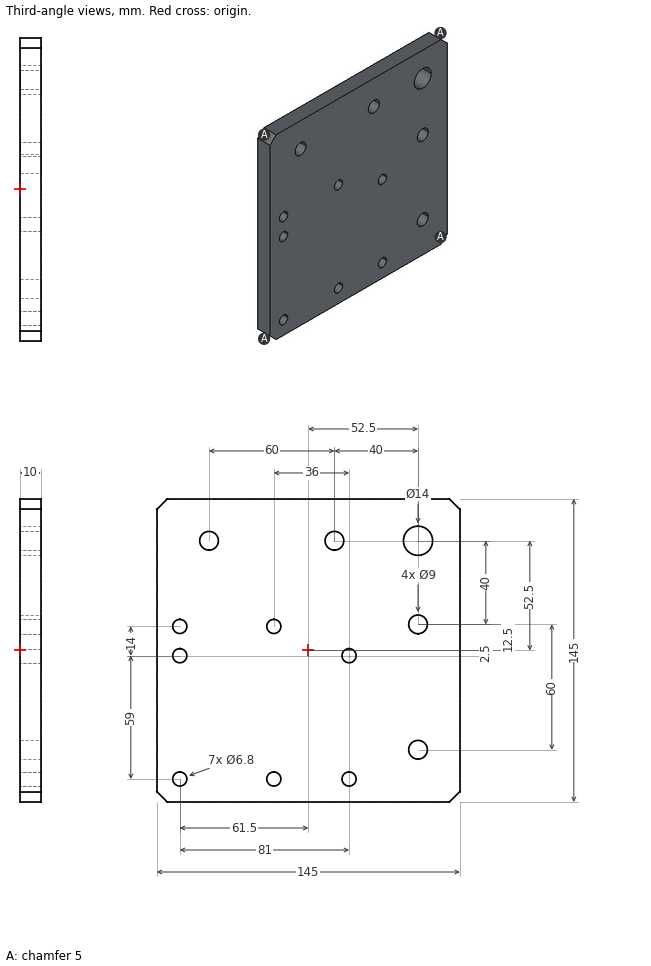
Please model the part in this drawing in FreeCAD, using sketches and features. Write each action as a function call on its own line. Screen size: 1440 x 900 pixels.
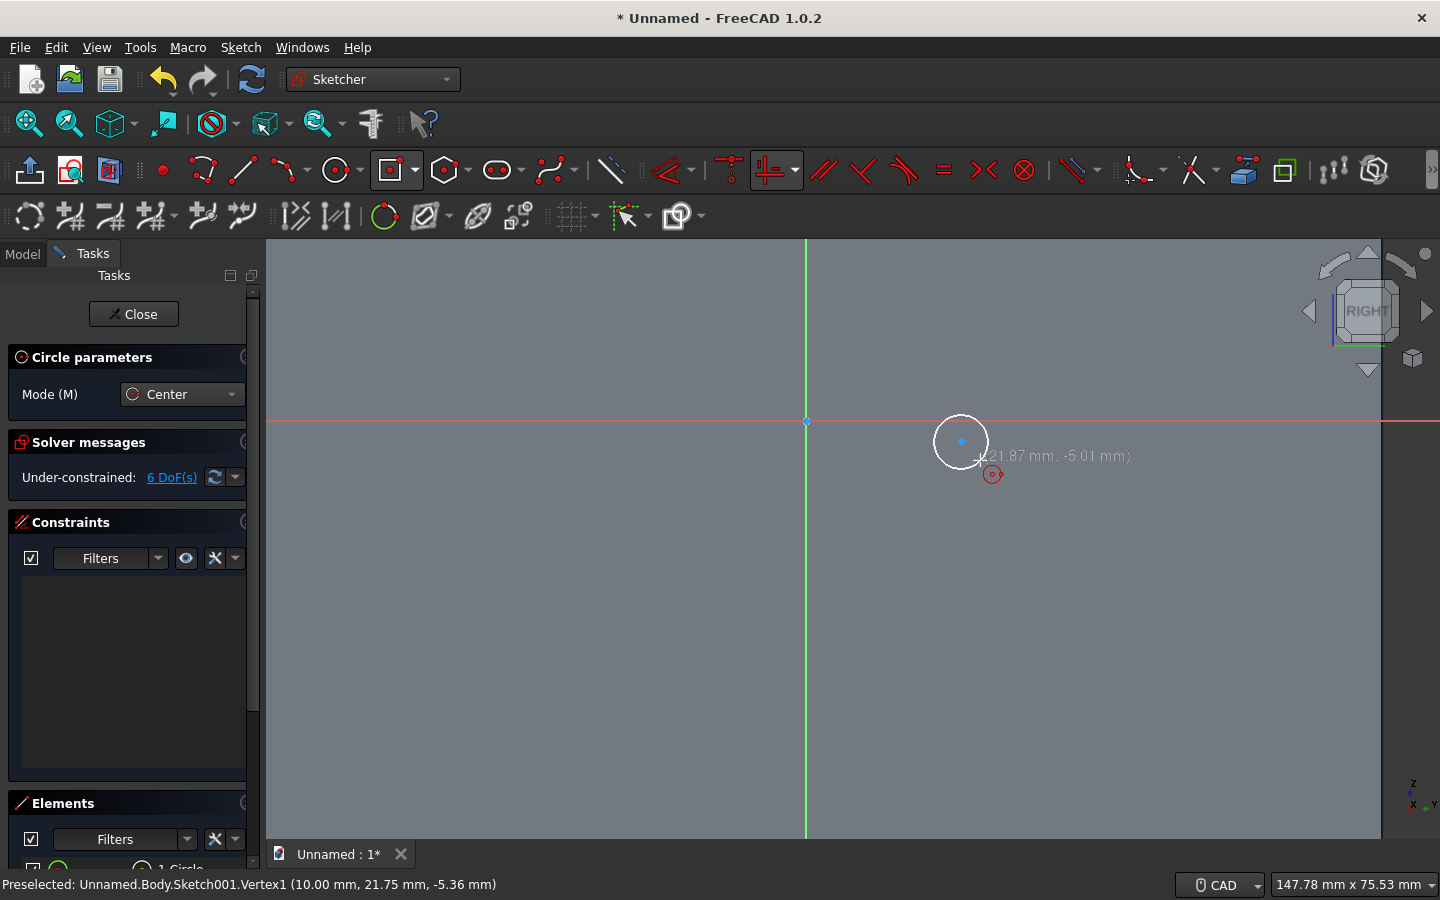
scroll(961, 441, down, 3)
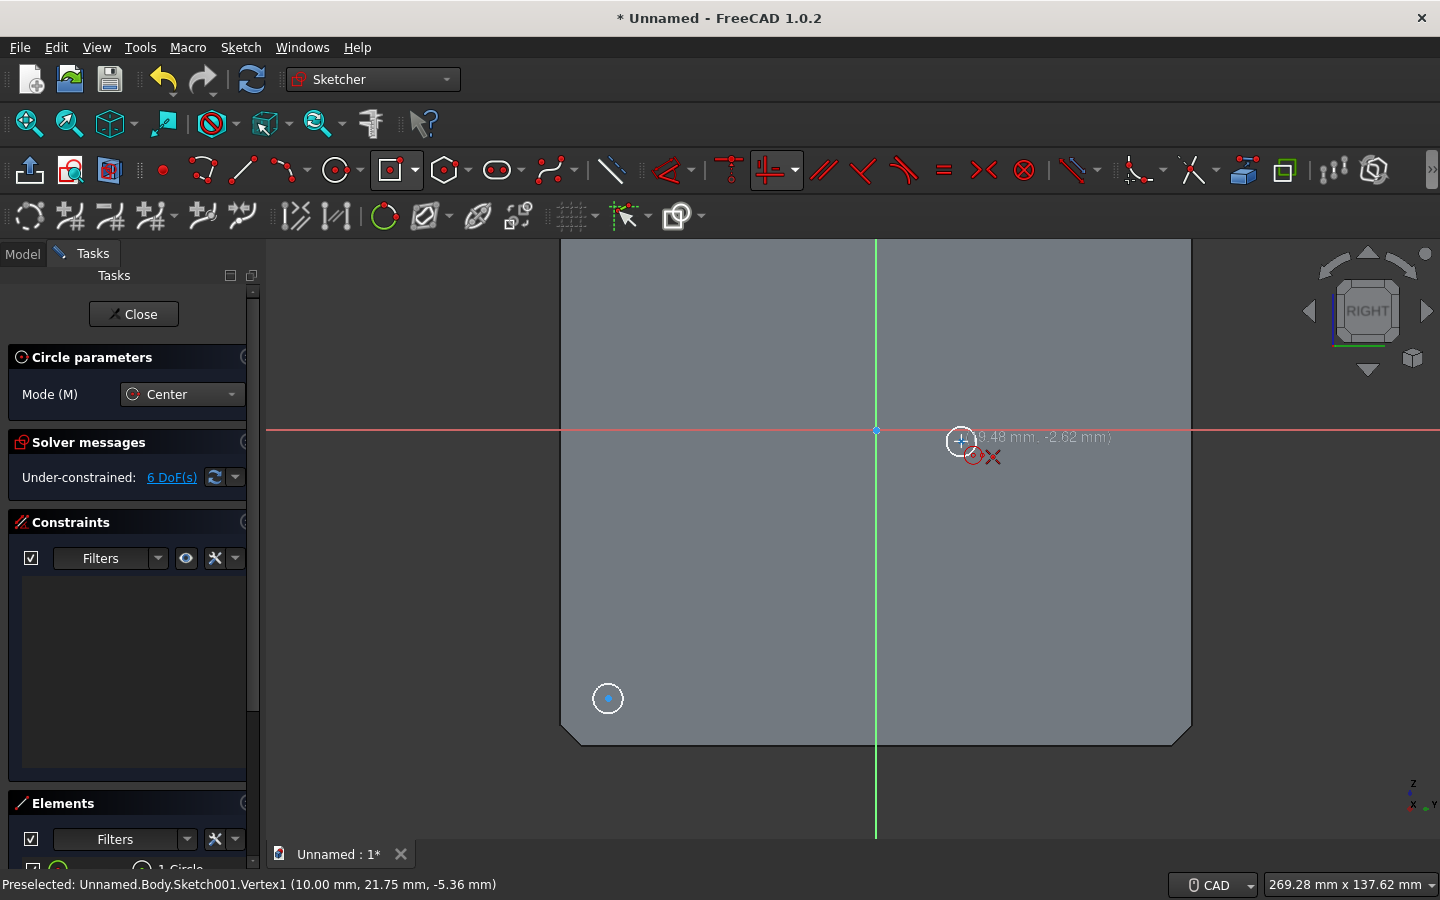
scroll(961, 698, up, 3)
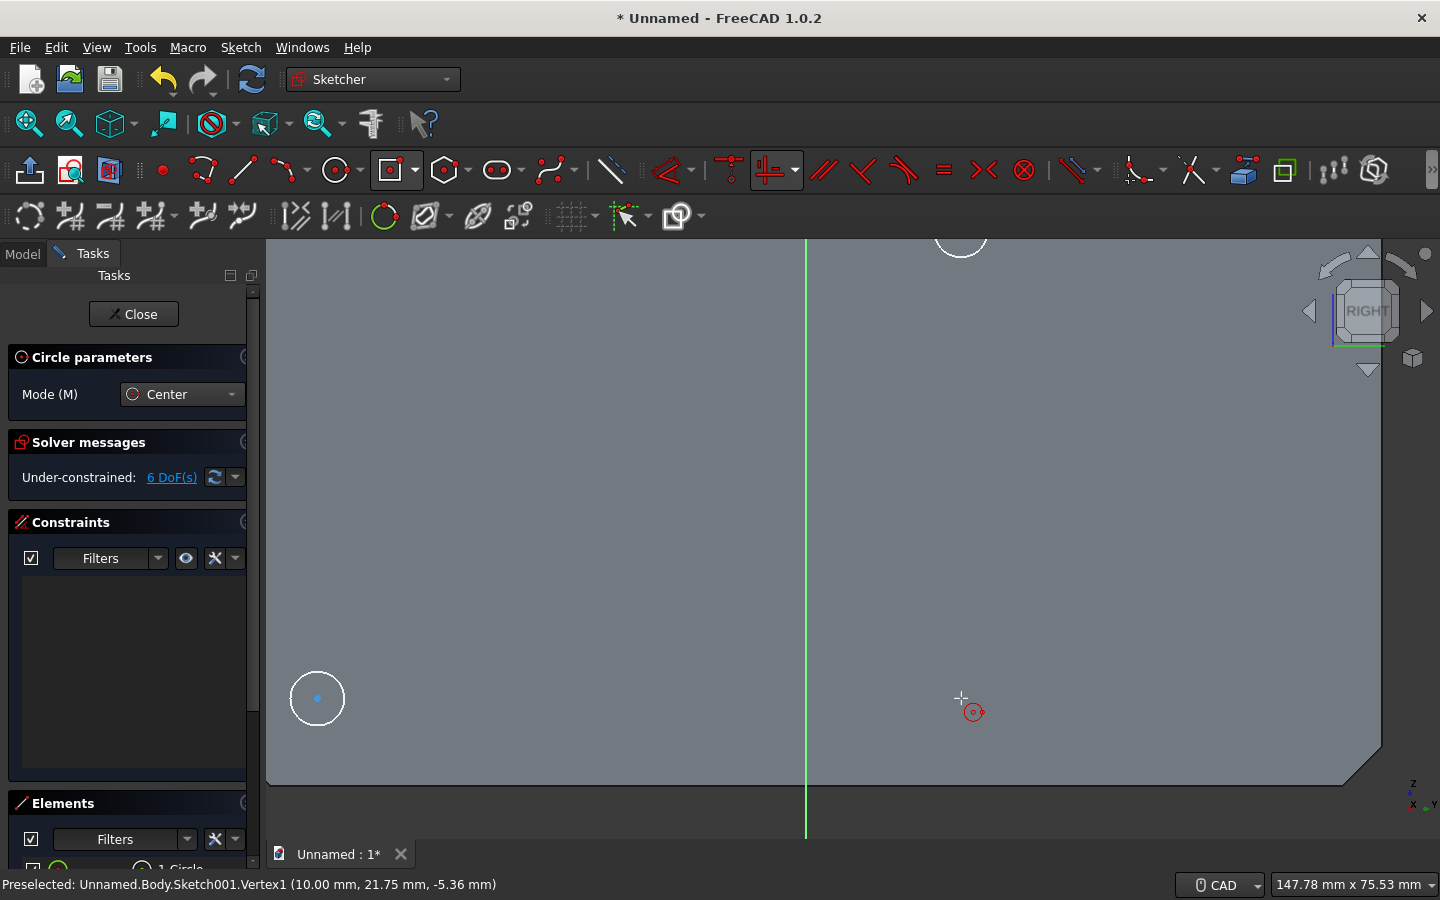
click(961, 698)
click(980, 679)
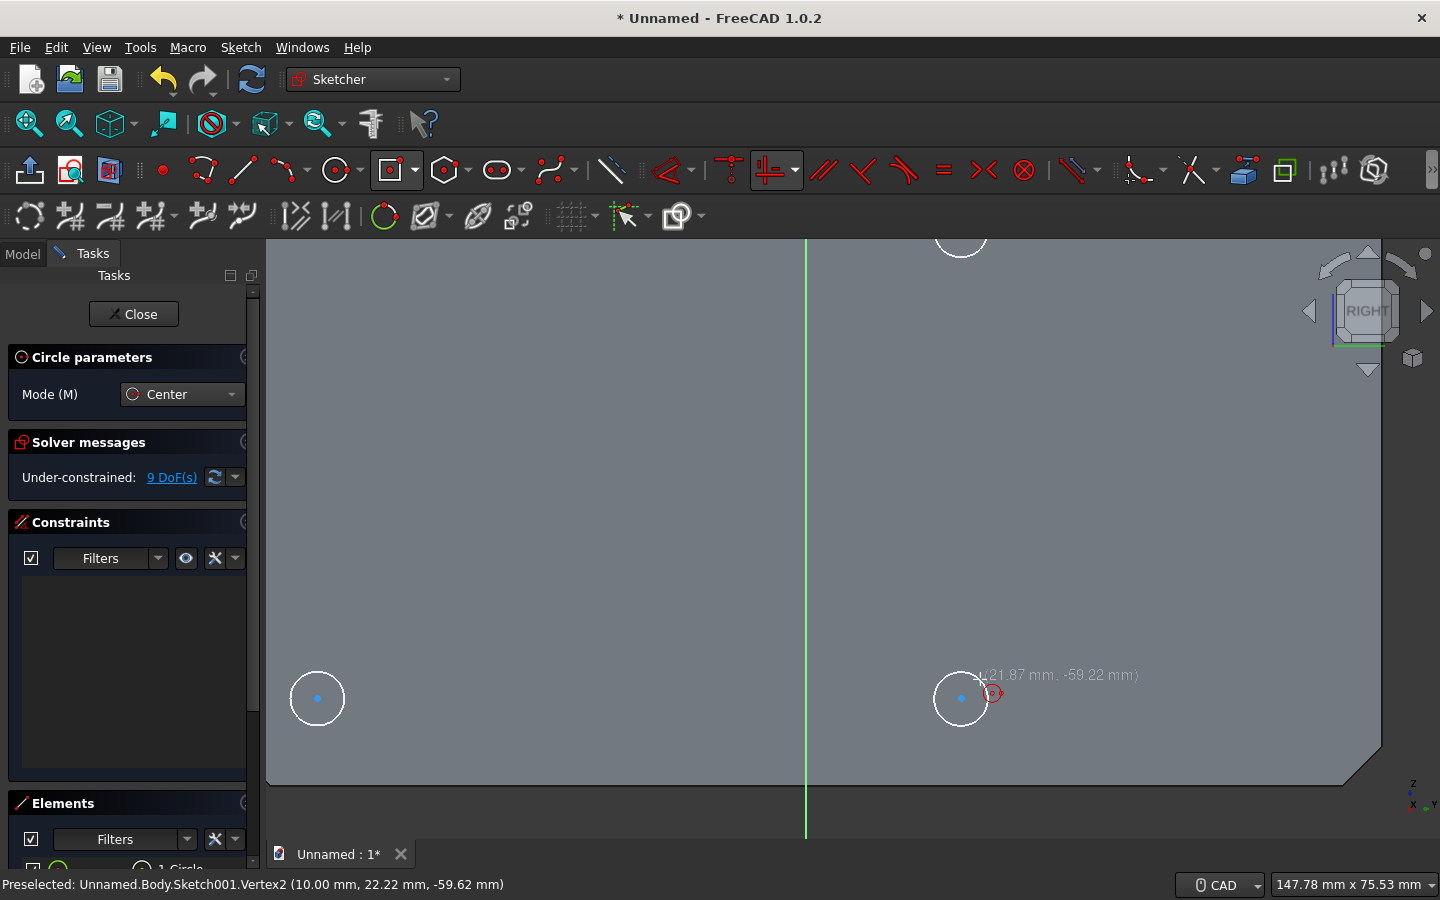
scroll(961, 698, down, 3)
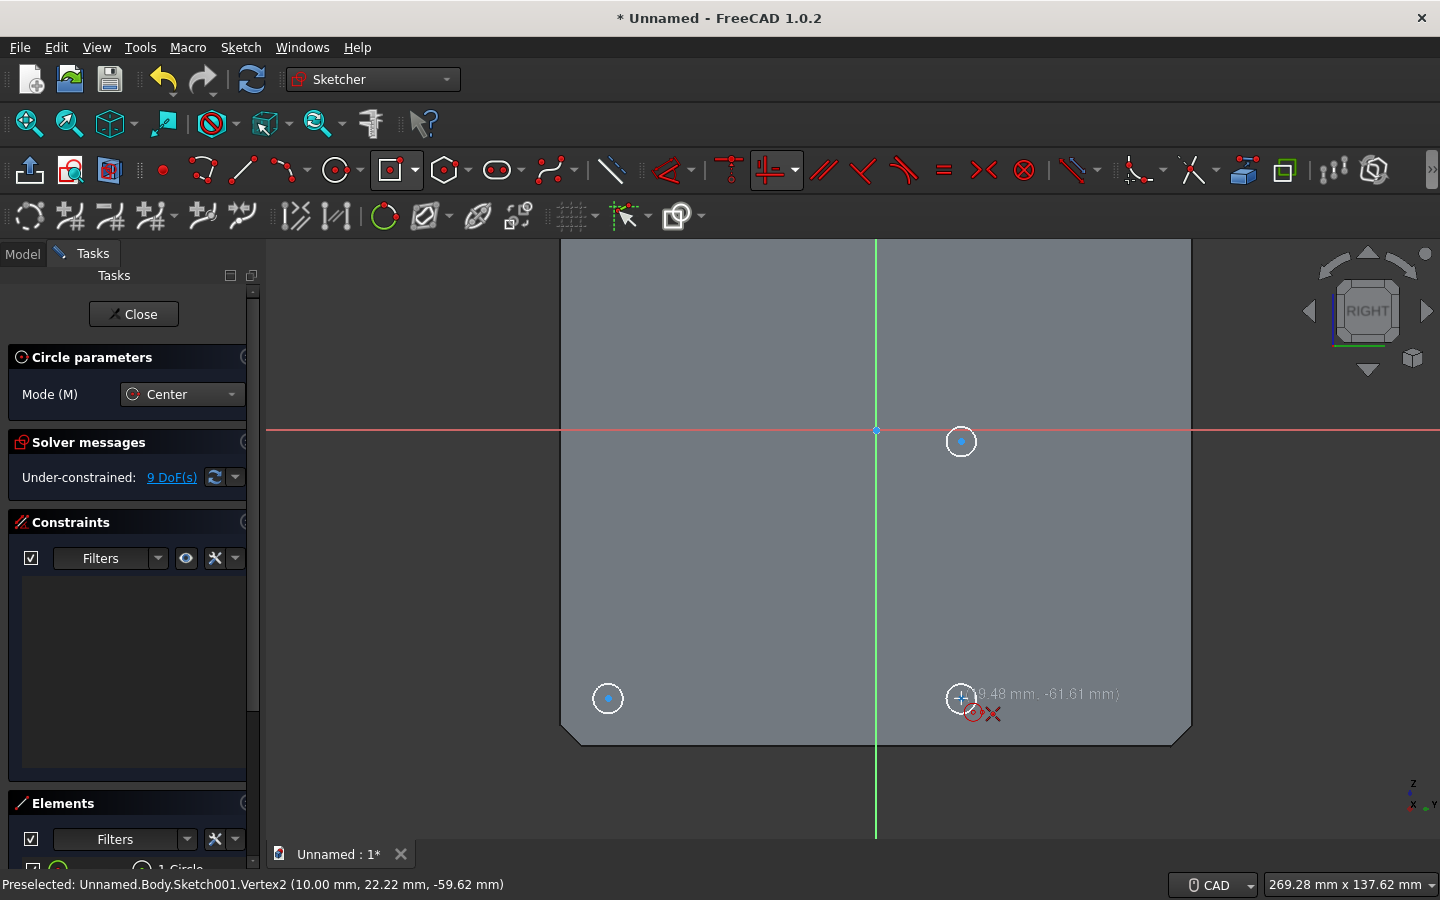
scroll(608, 441, up, 3)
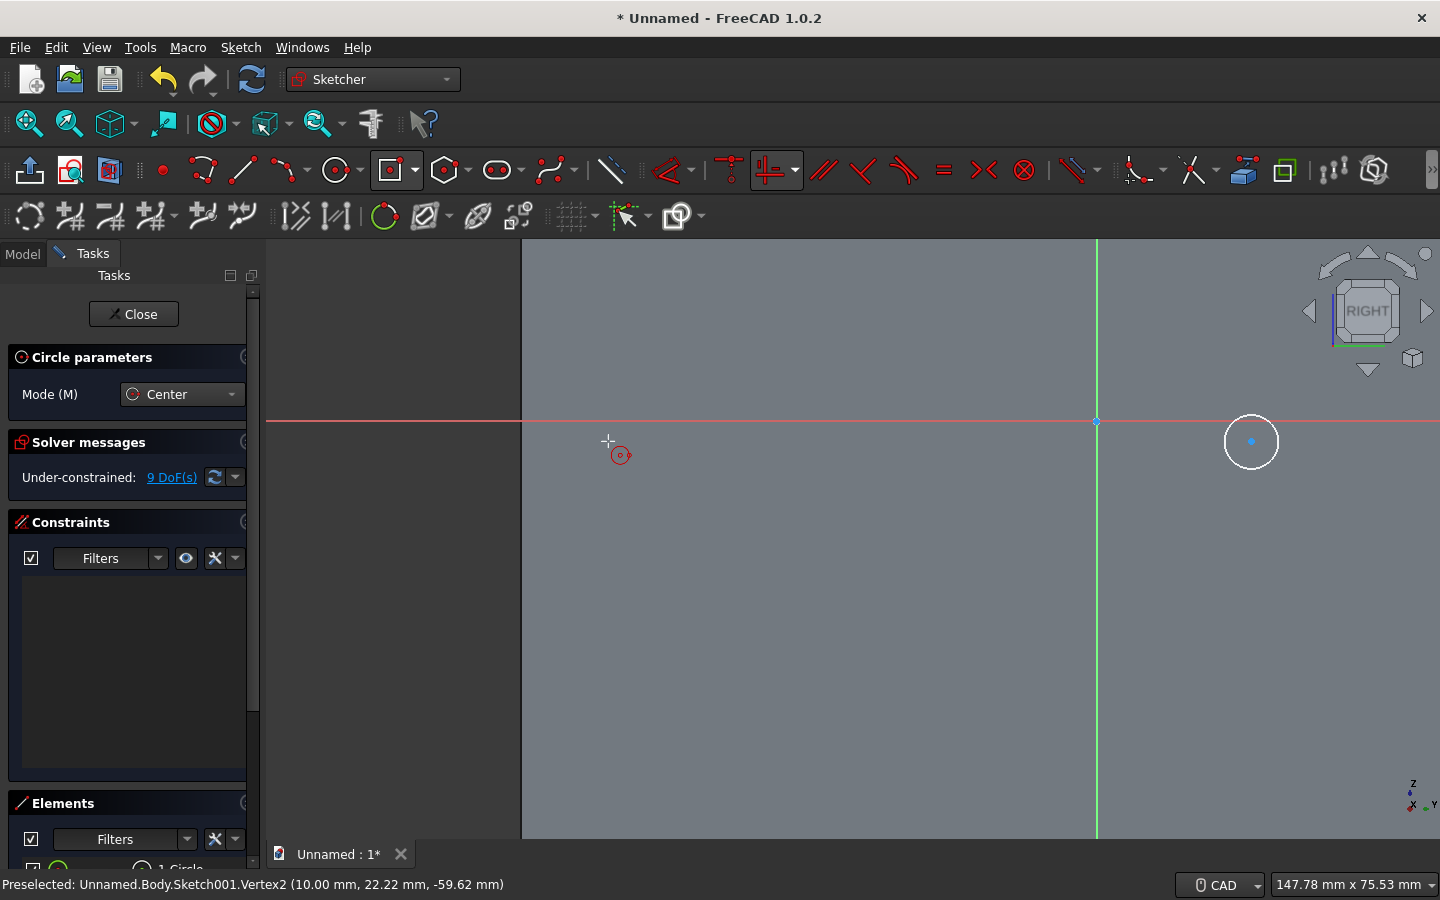
click(608, 441)
click(627, 460)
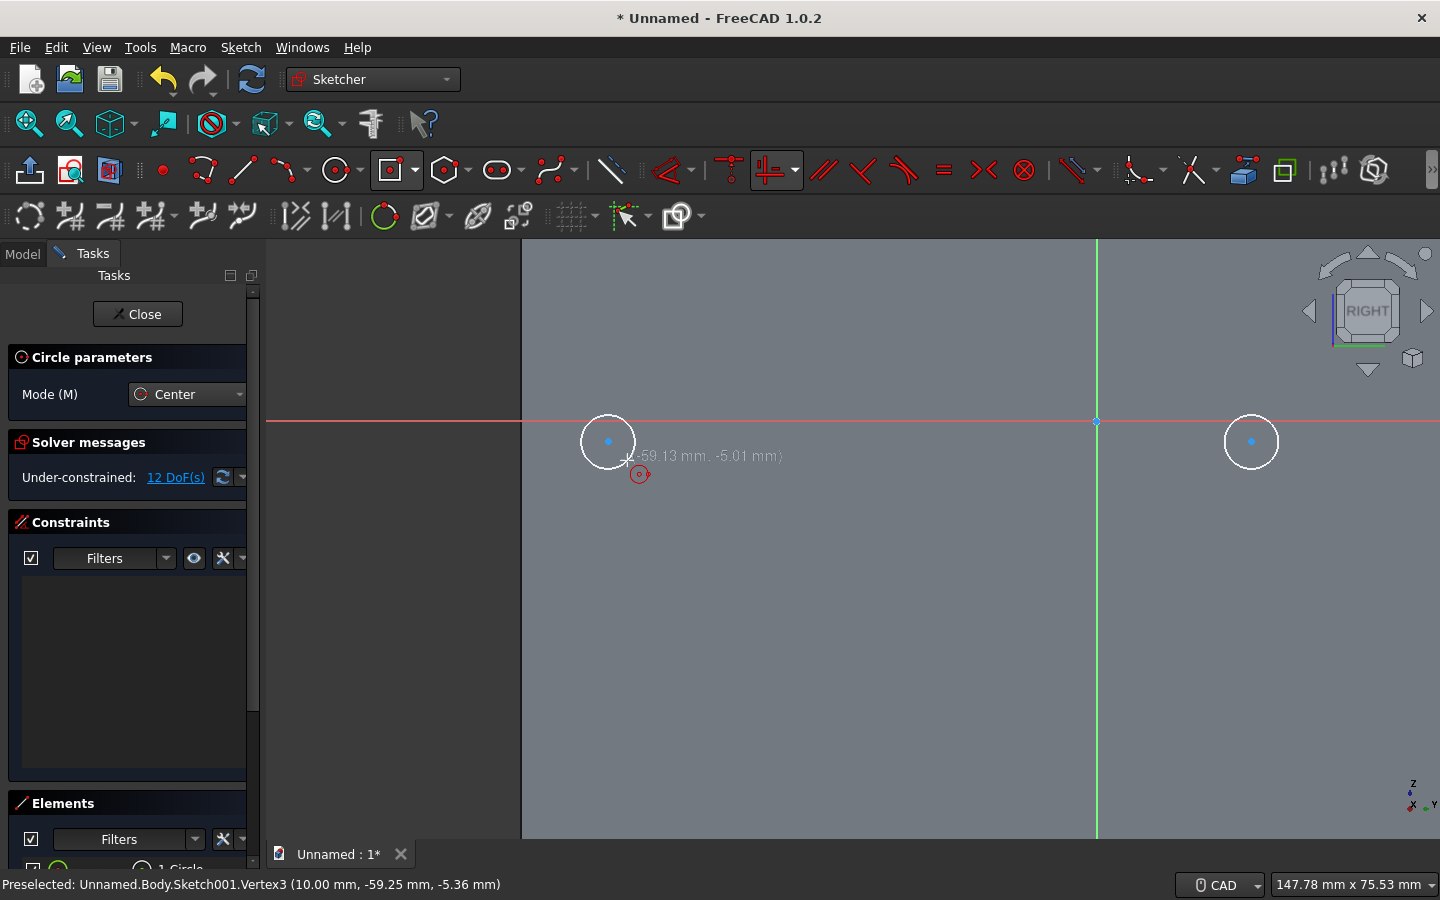
click(608, 330)
click(627, 311)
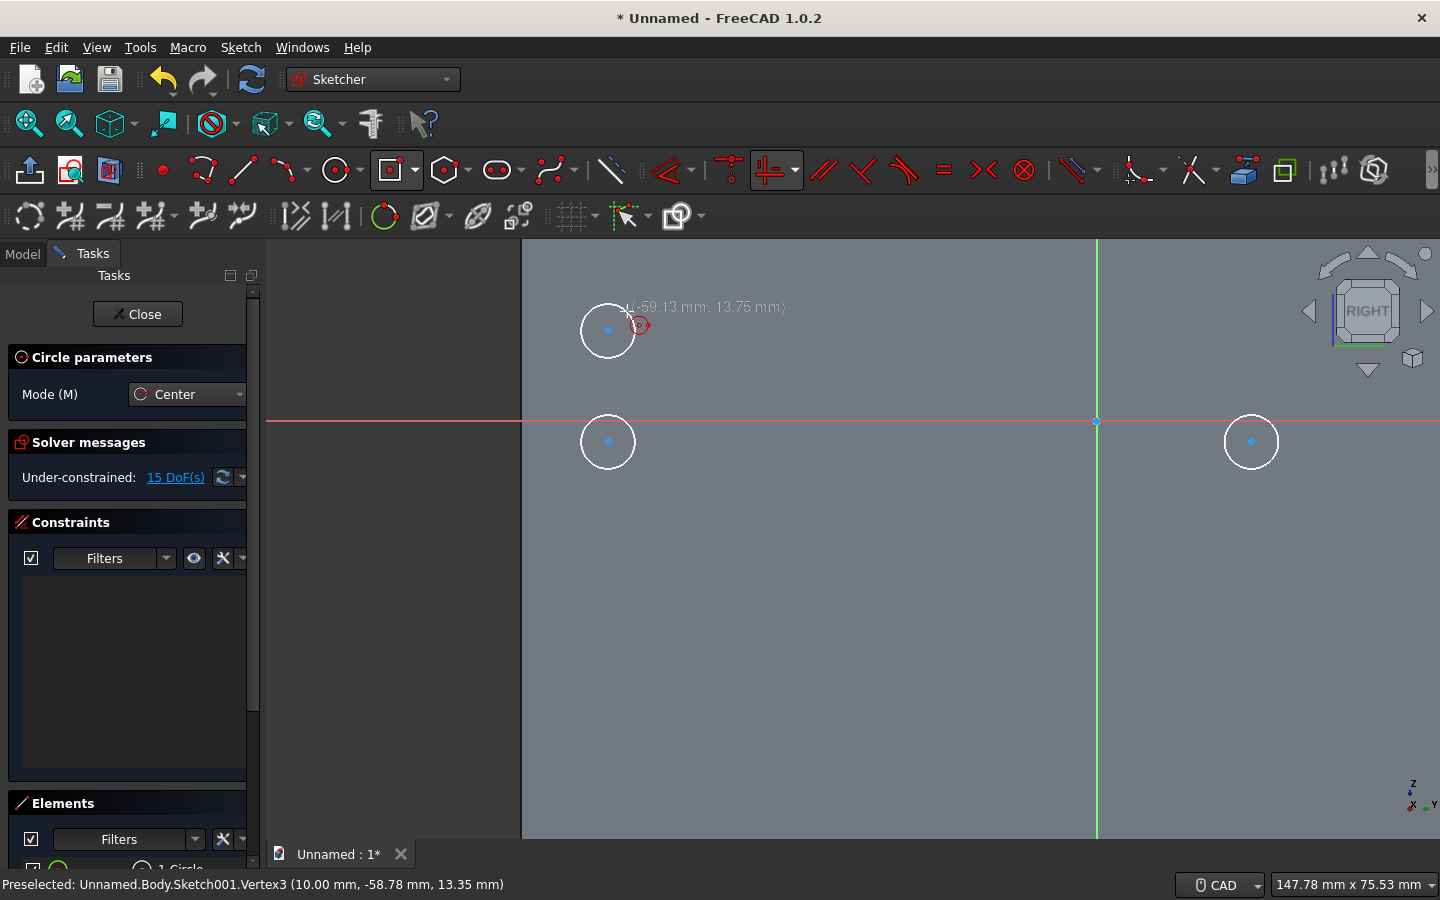
click(966, 330)
click(985, 311)